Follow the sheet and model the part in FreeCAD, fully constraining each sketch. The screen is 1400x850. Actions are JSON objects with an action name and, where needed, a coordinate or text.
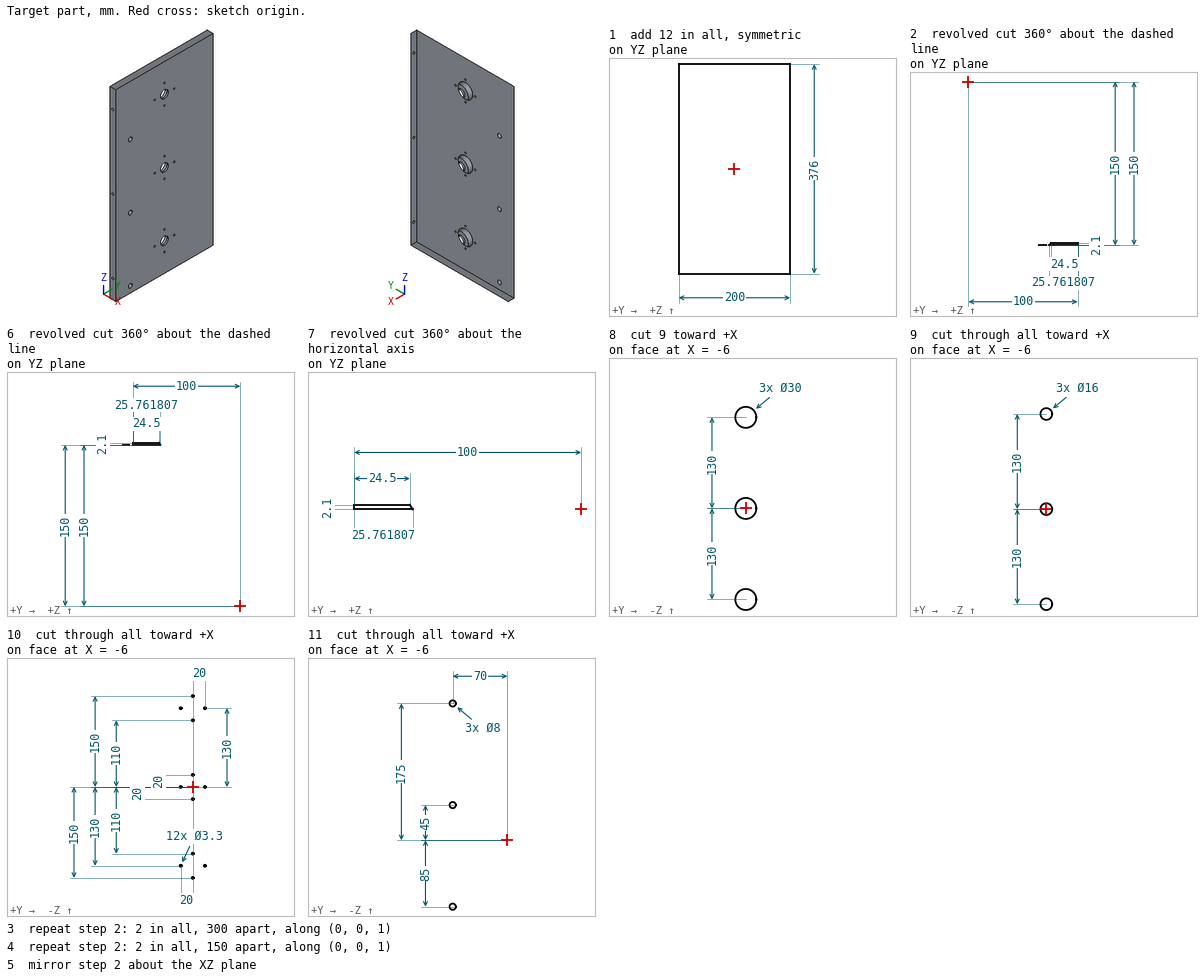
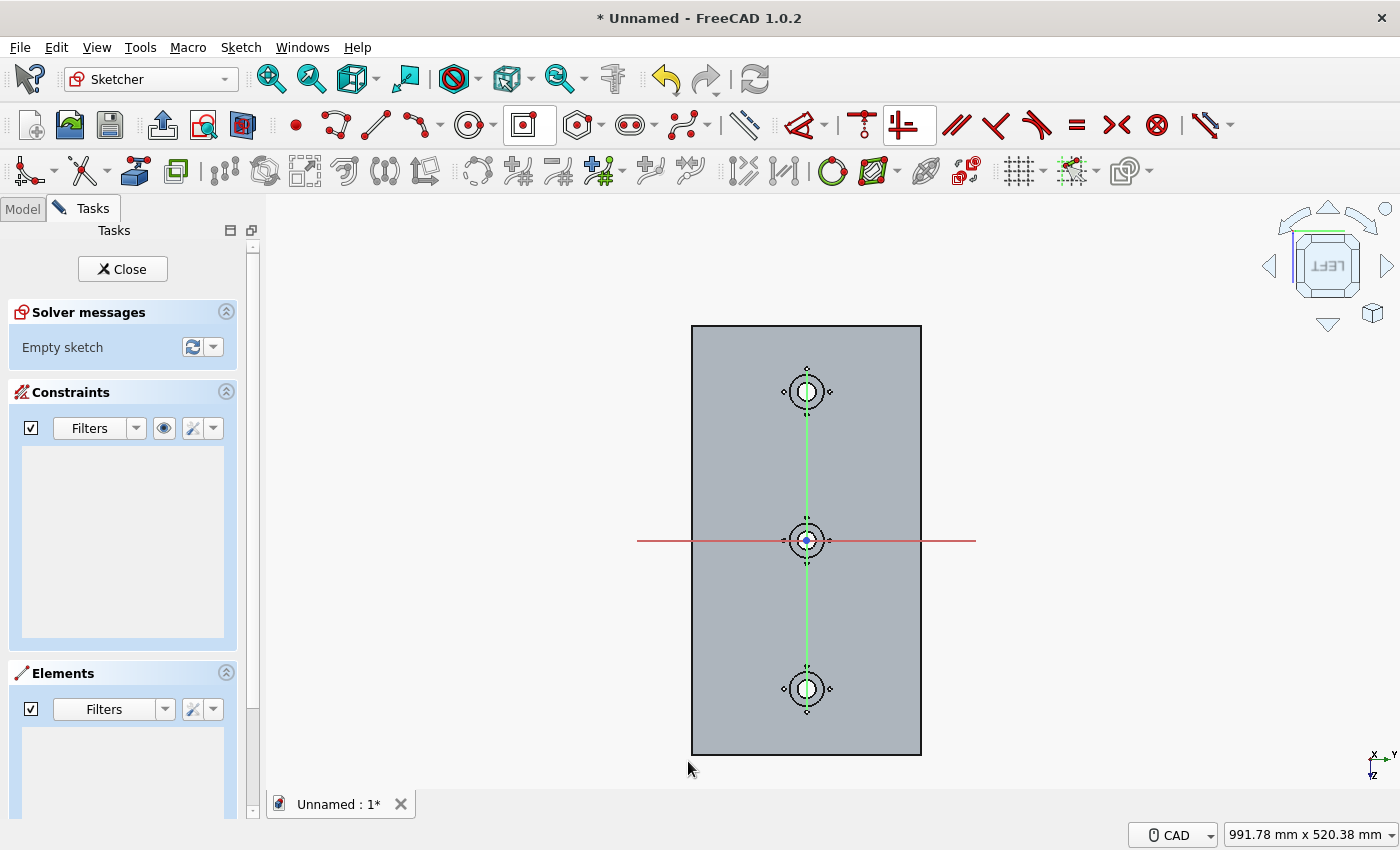
{"action": "left_click", "coordinate": [470, 126]}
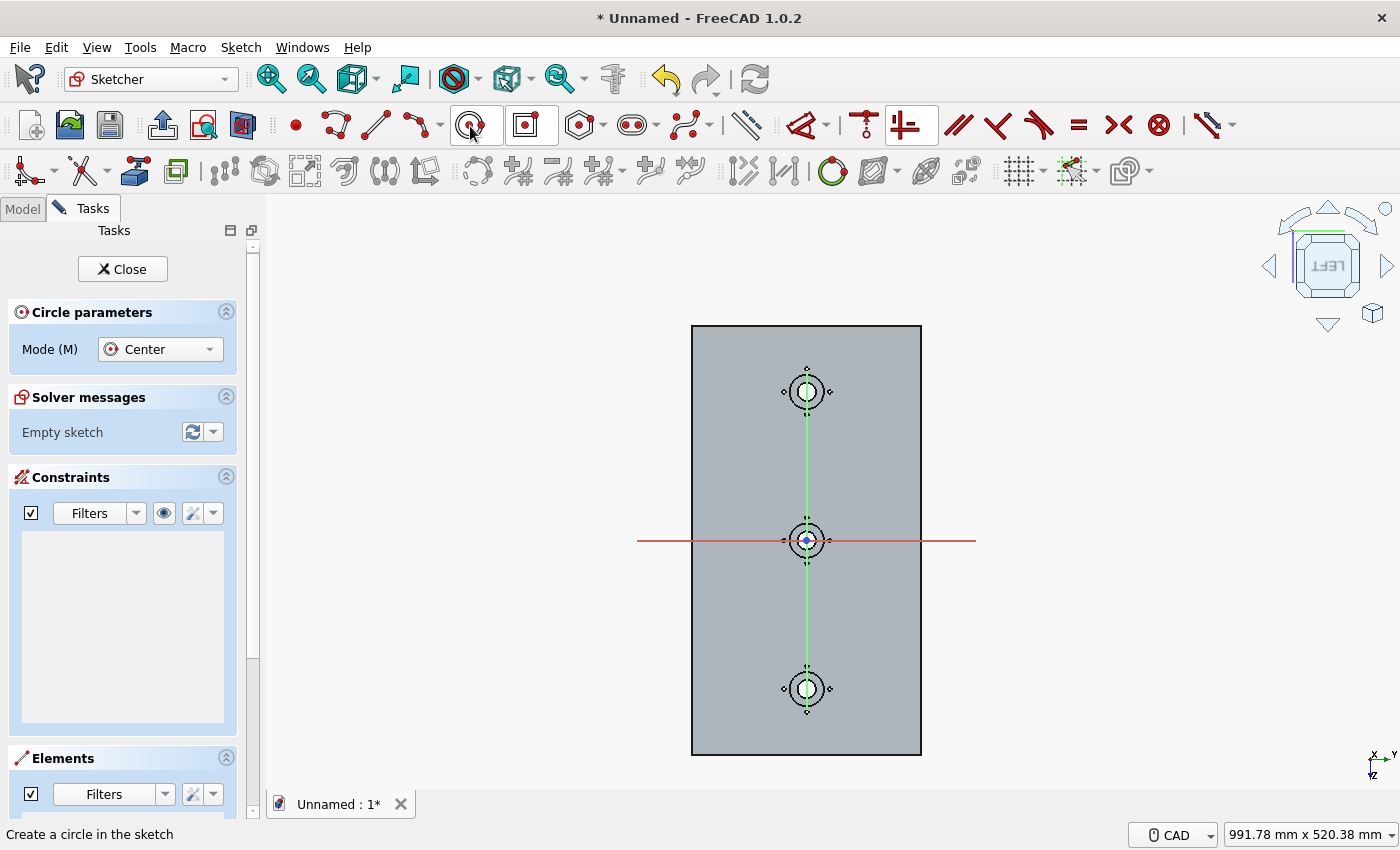
{"action": "scroll", "coordinate": [727, 340], "scroll_direction": "up", "scroll_amount": 9}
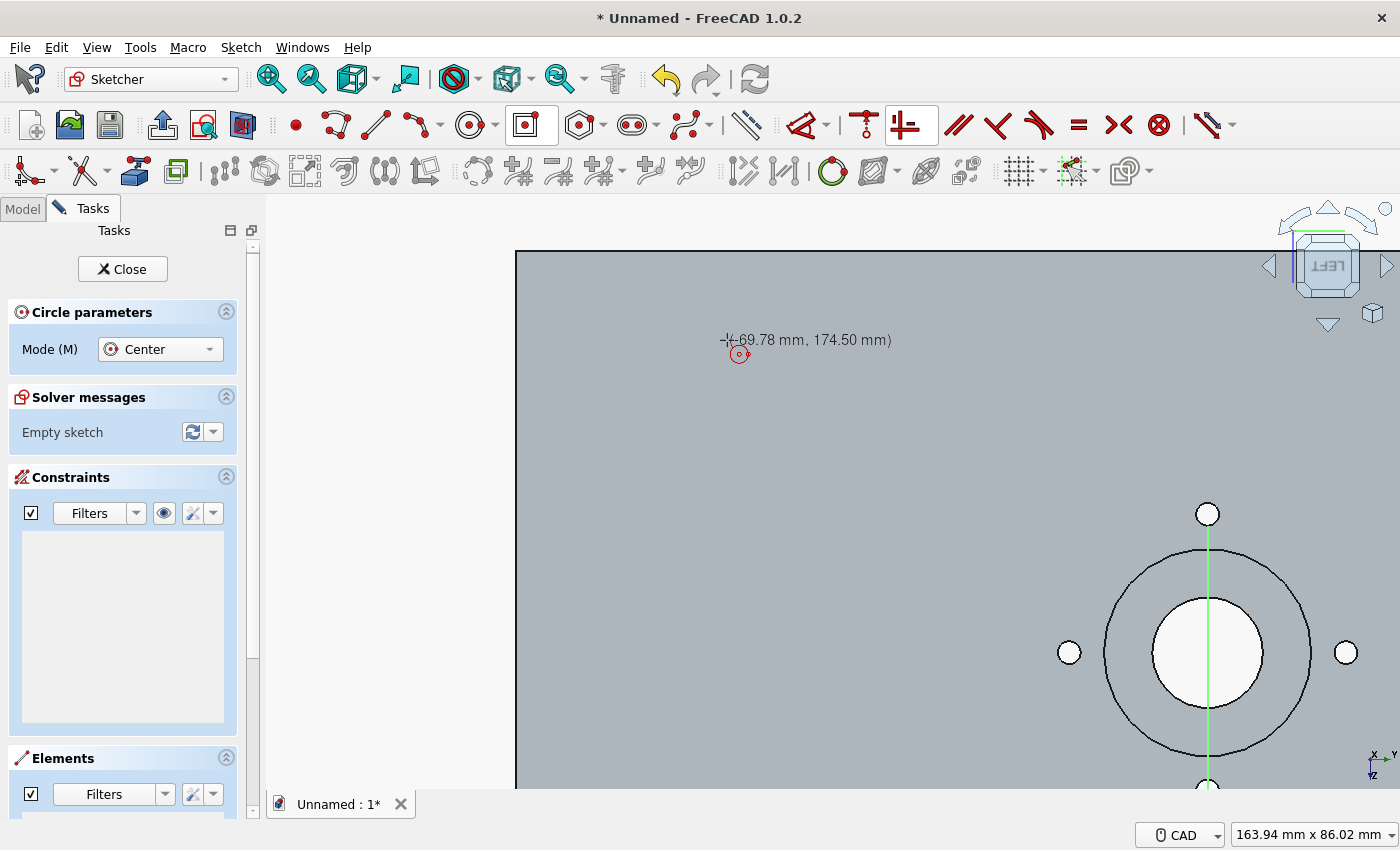
{"action": "scroll", "coordinate": [717, 302], "scroll_direction": "down", "scroll_amount": 8}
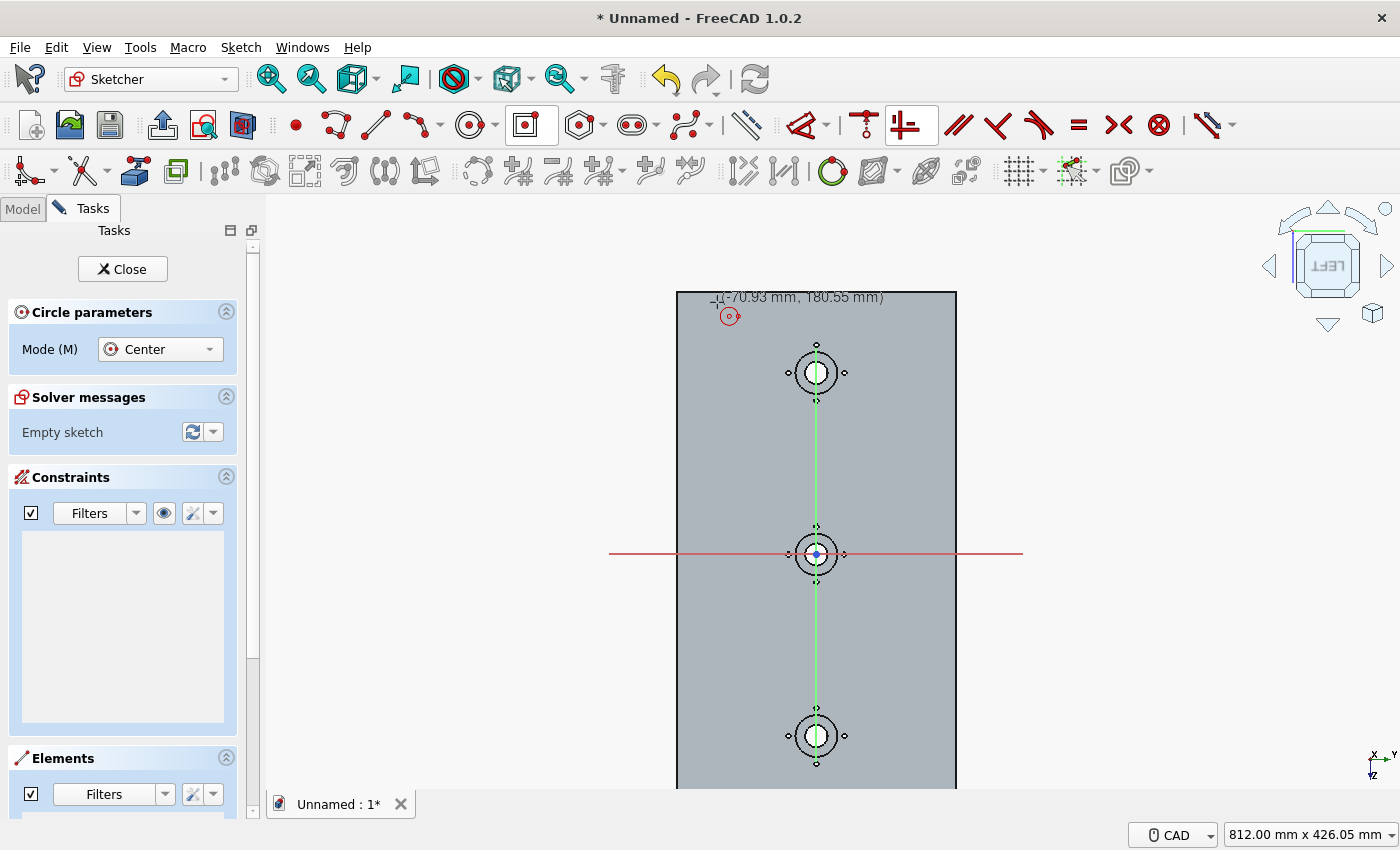
{"action": "left_click", "coordinate": [719, 310]}
{"action": "mouse_move", "coordinate": [723, 306]}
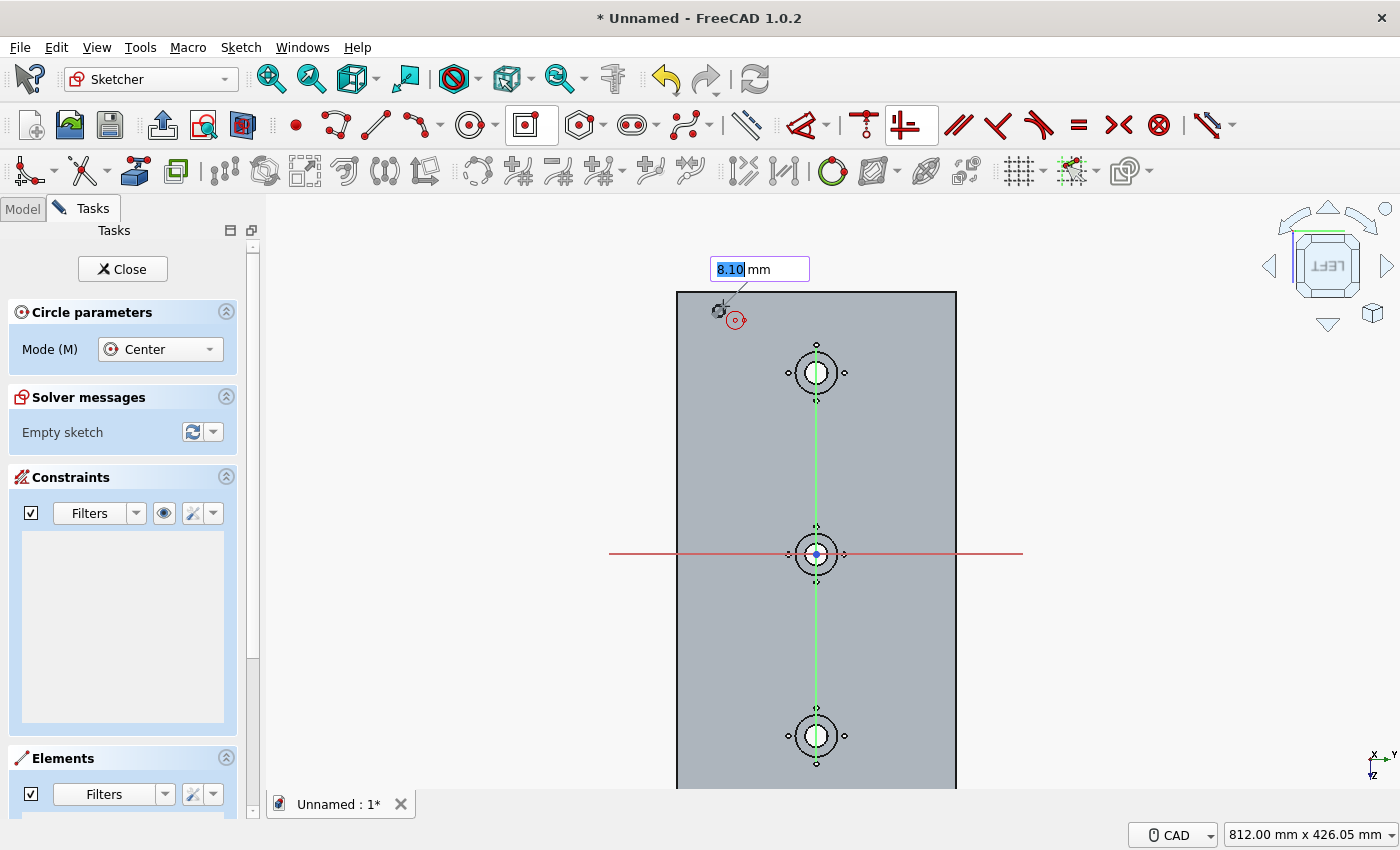
{"action": "type", "text": "8"}
{"action": "key", "text": "Return"}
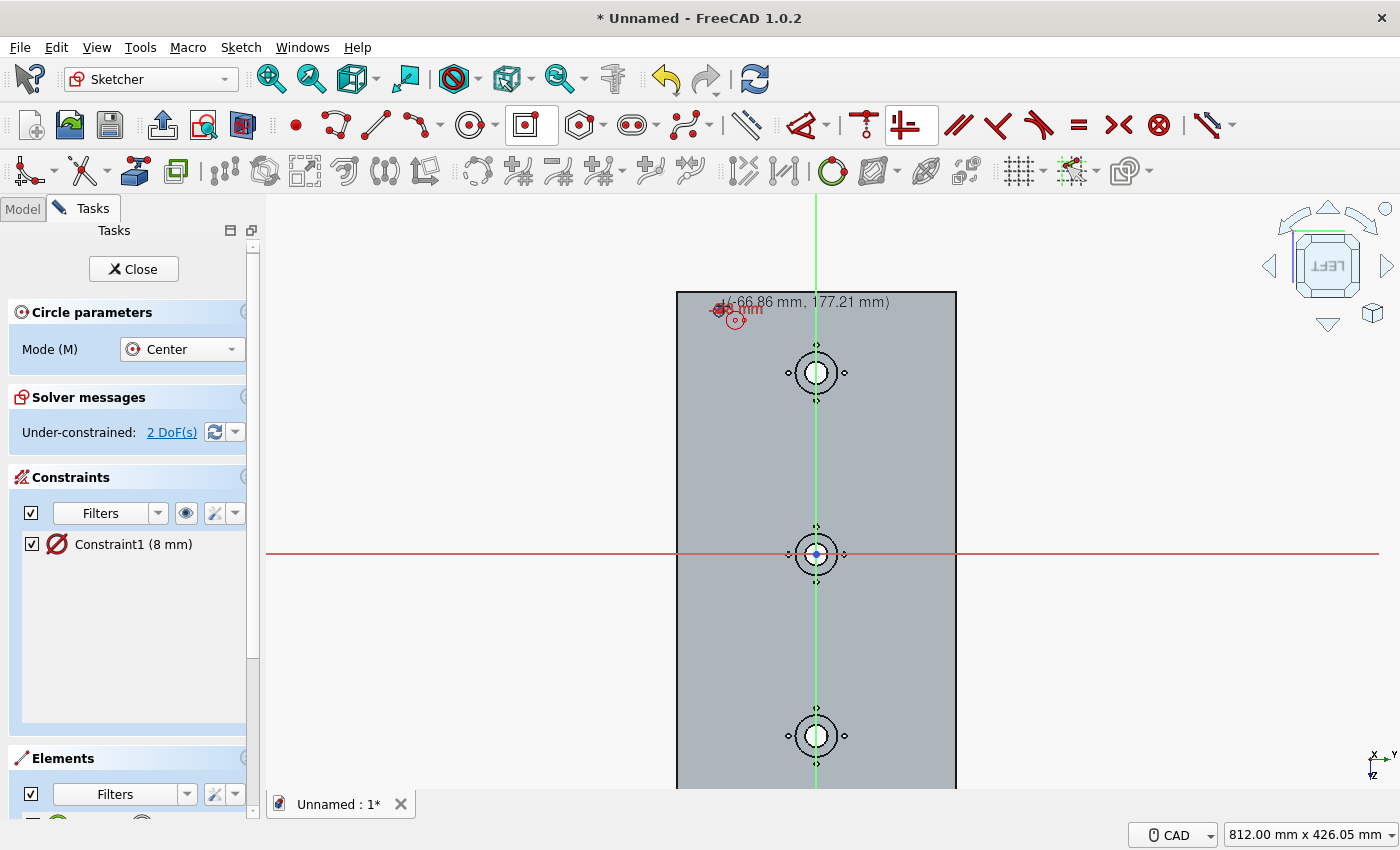
{"action": "scroll", "coordinate": [719, 492], "scroll_direction": "up", "scroll_amount": 8}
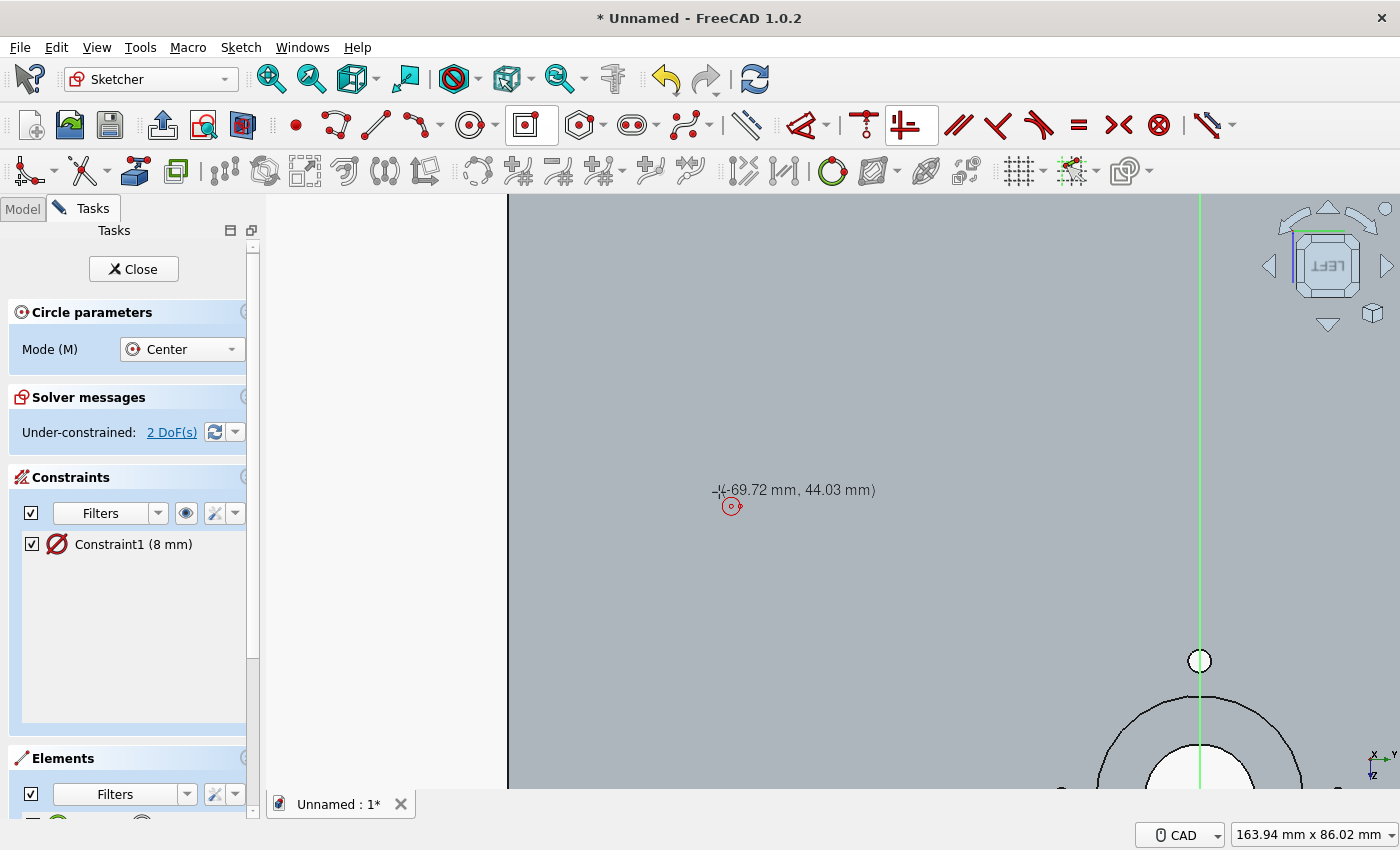
{"action": "scroll", "coordinate": [719, 492], "scroll_direction": "down", "scroll_amount": 8}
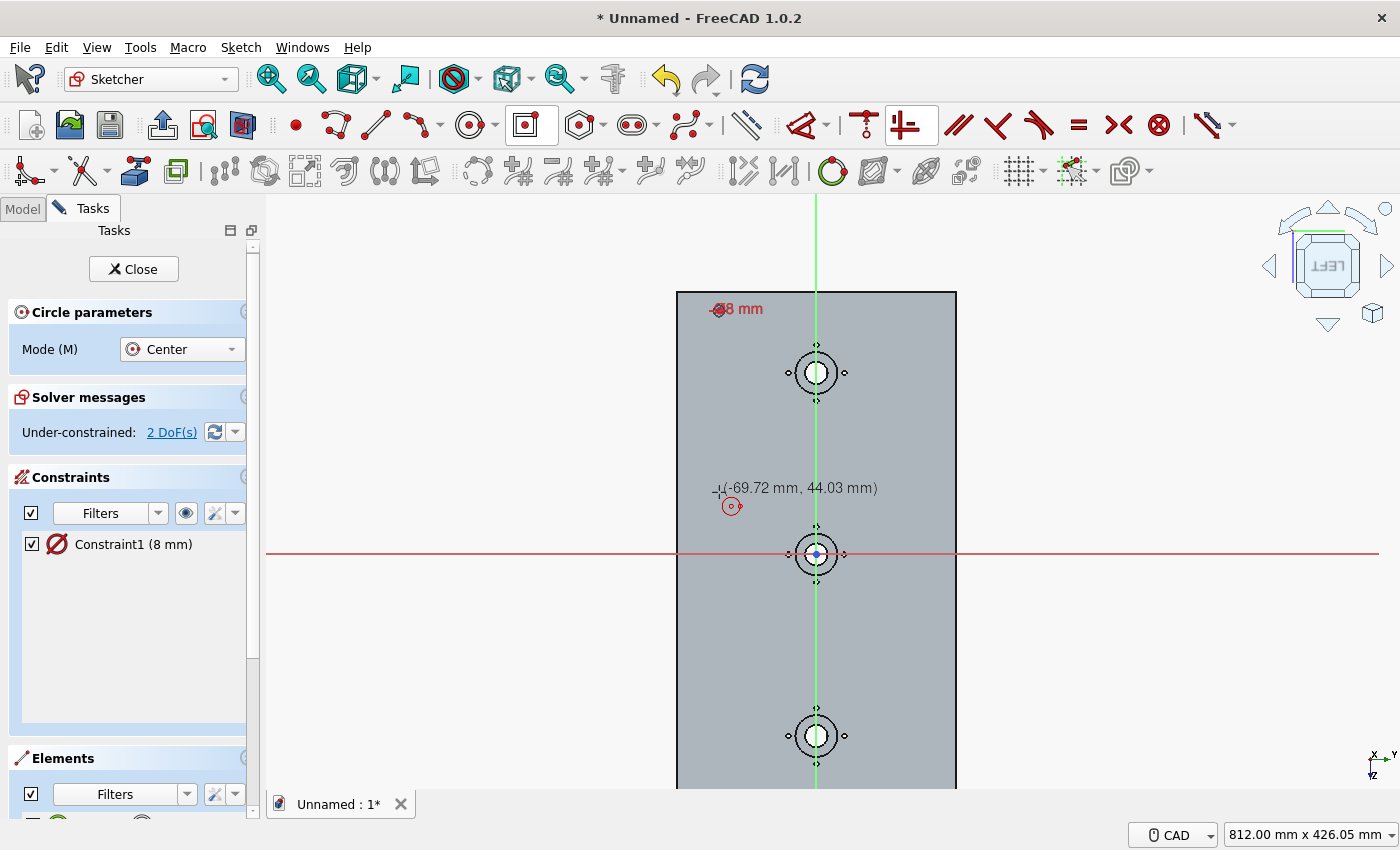
{"action": "left_click", "coordinate": [719, 492]}
{"action": "mouse_move", "coordinate": [723, 488]}